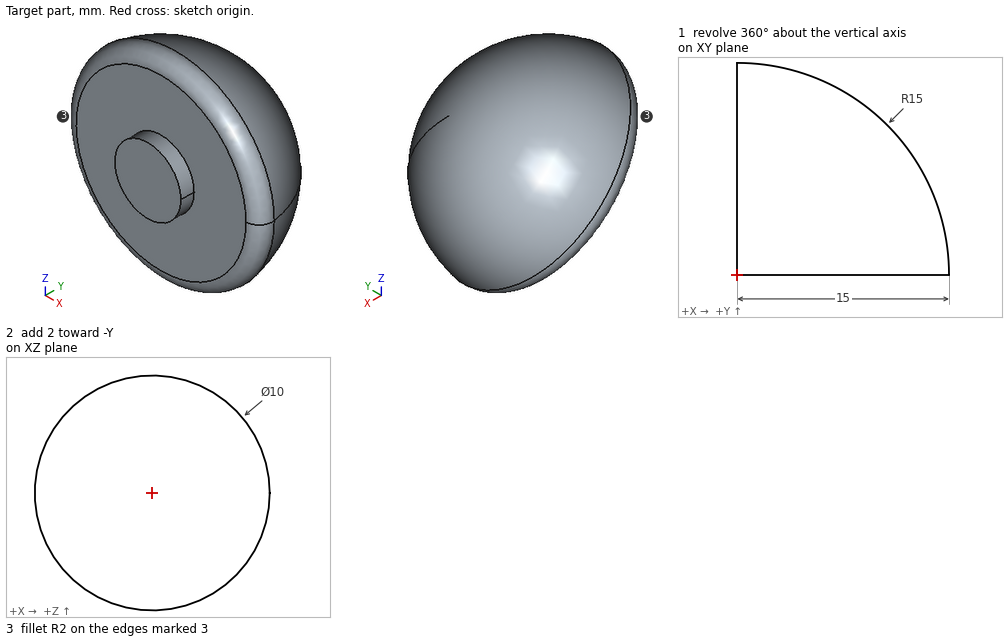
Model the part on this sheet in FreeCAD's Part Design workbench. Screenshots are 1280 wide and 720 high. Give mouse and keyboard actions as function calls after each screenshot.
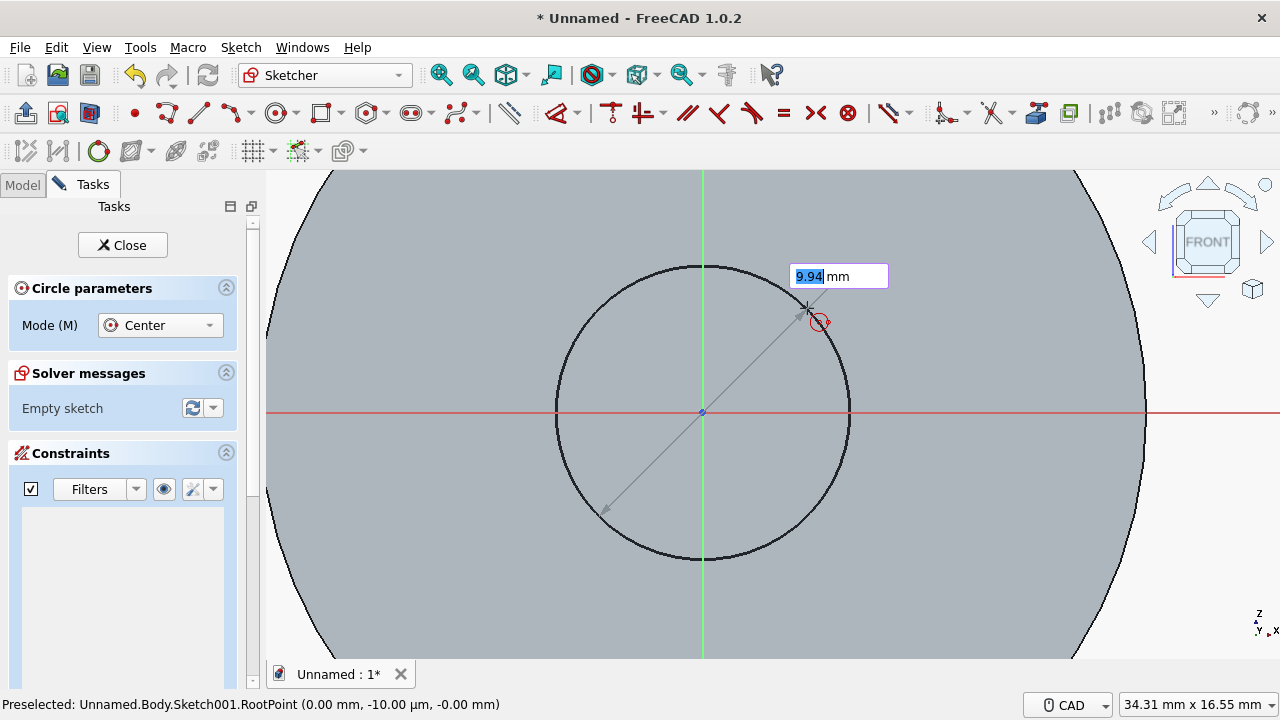
text(10)
key(Return)
key(Escape)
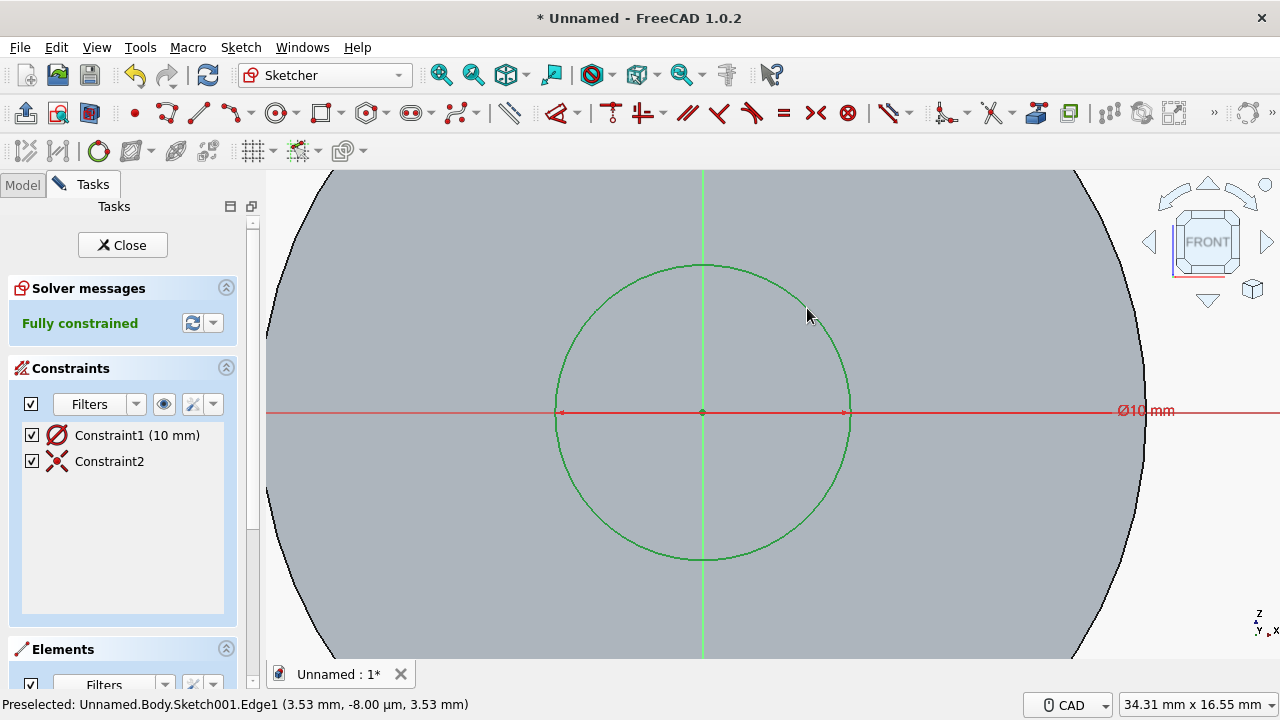
click(123, 245)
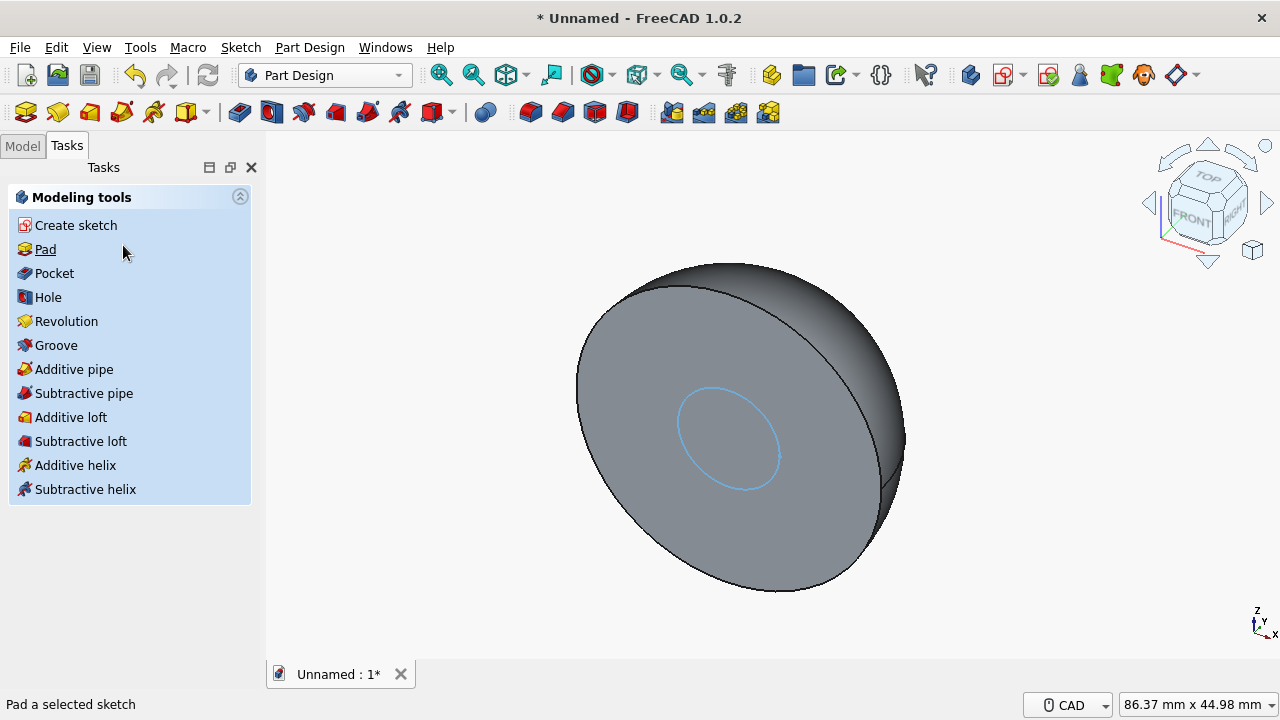
click(26, 112)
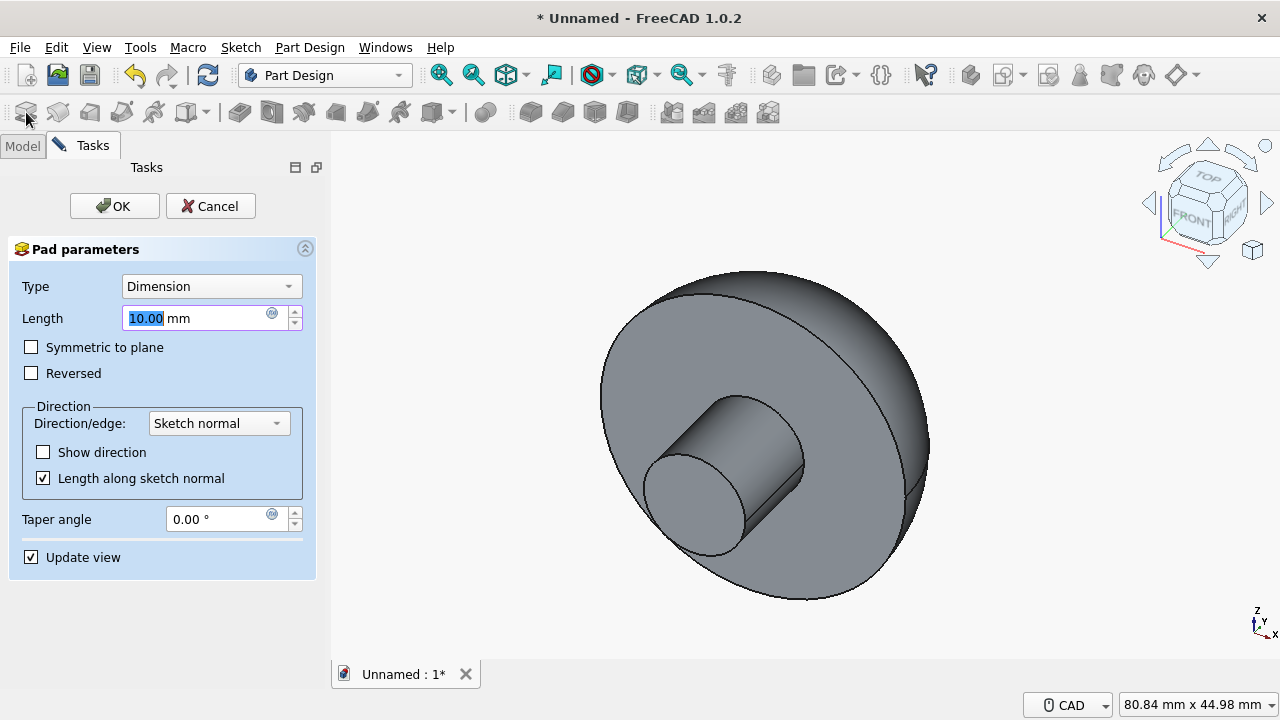
text(2)
key(Tab)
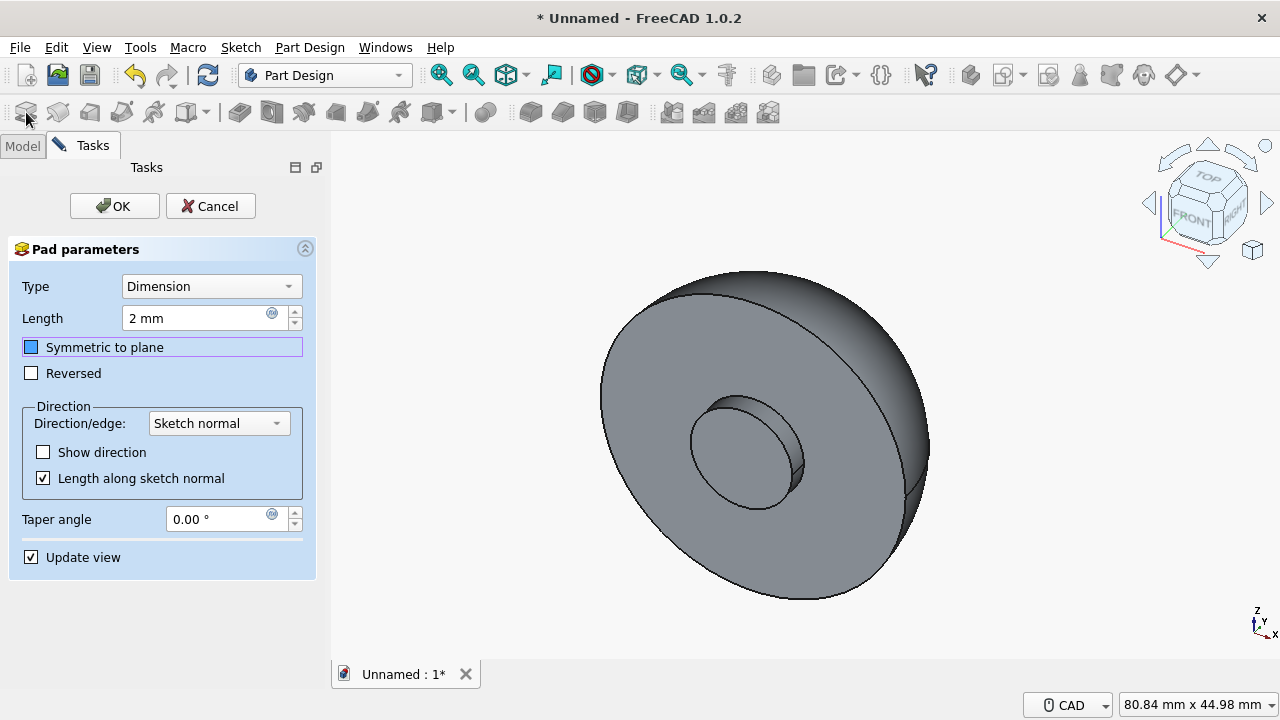
click(115, 206)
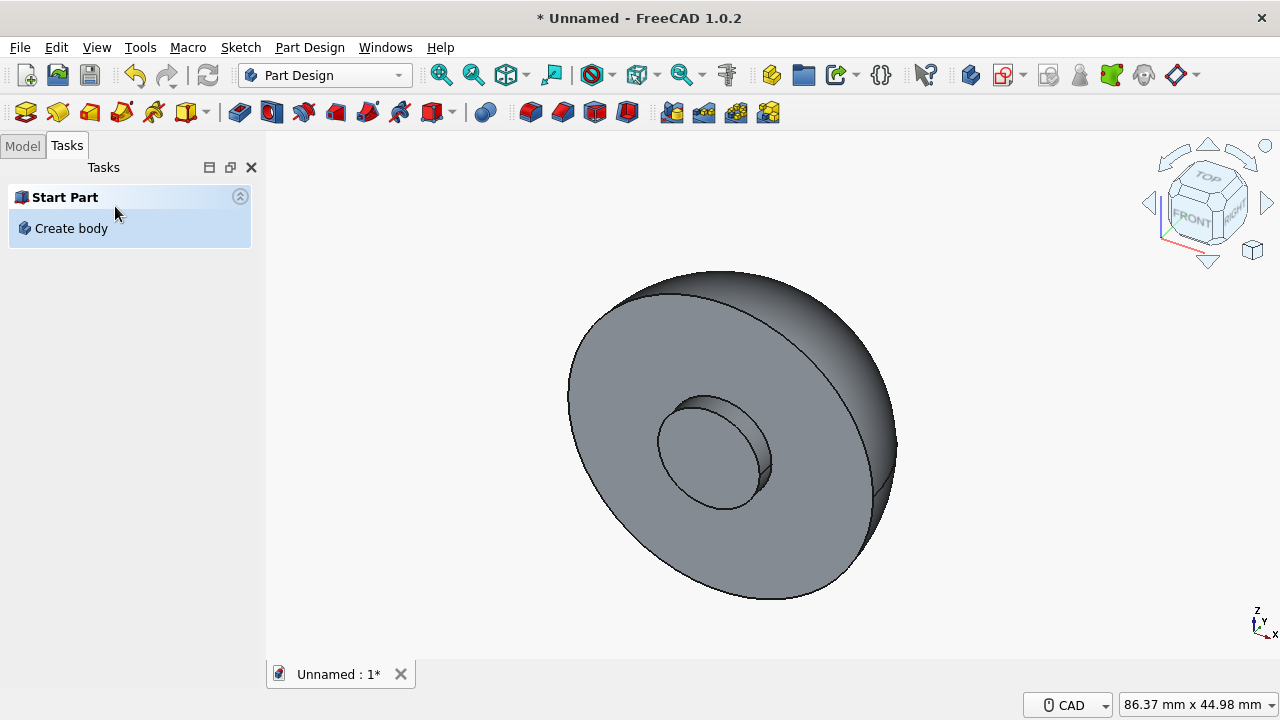
click(597, 320)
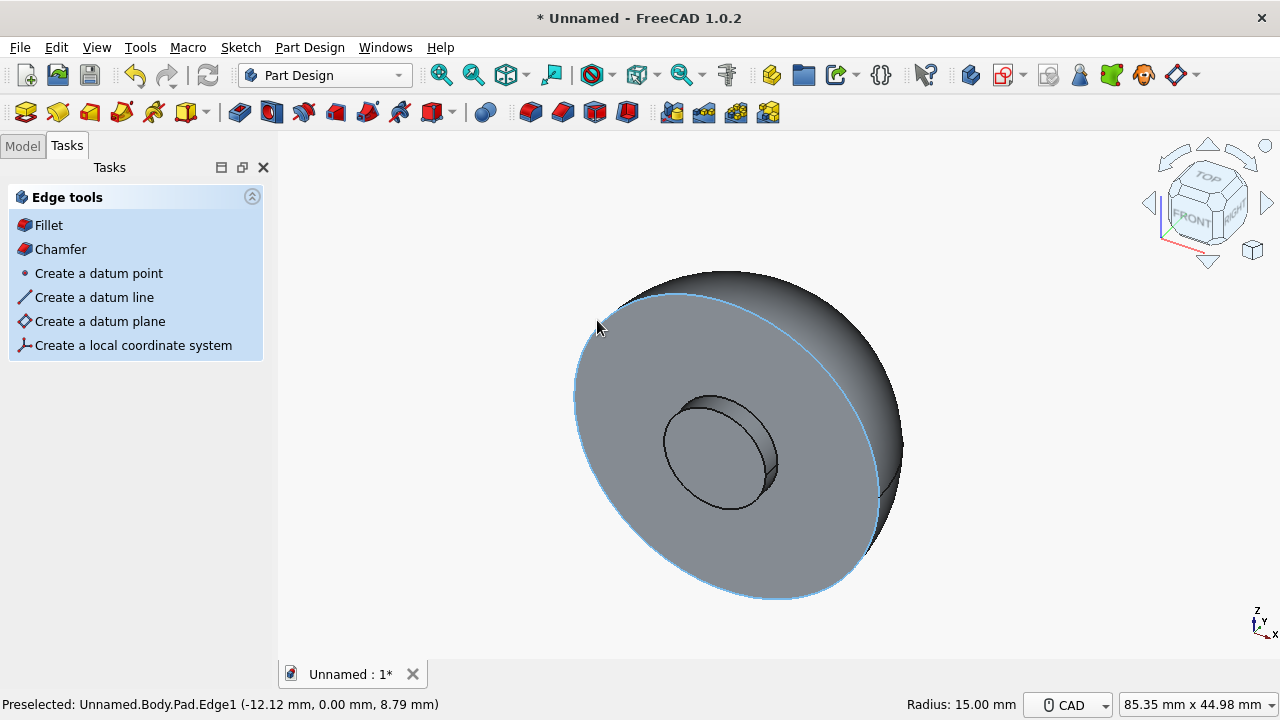
click(532, 112)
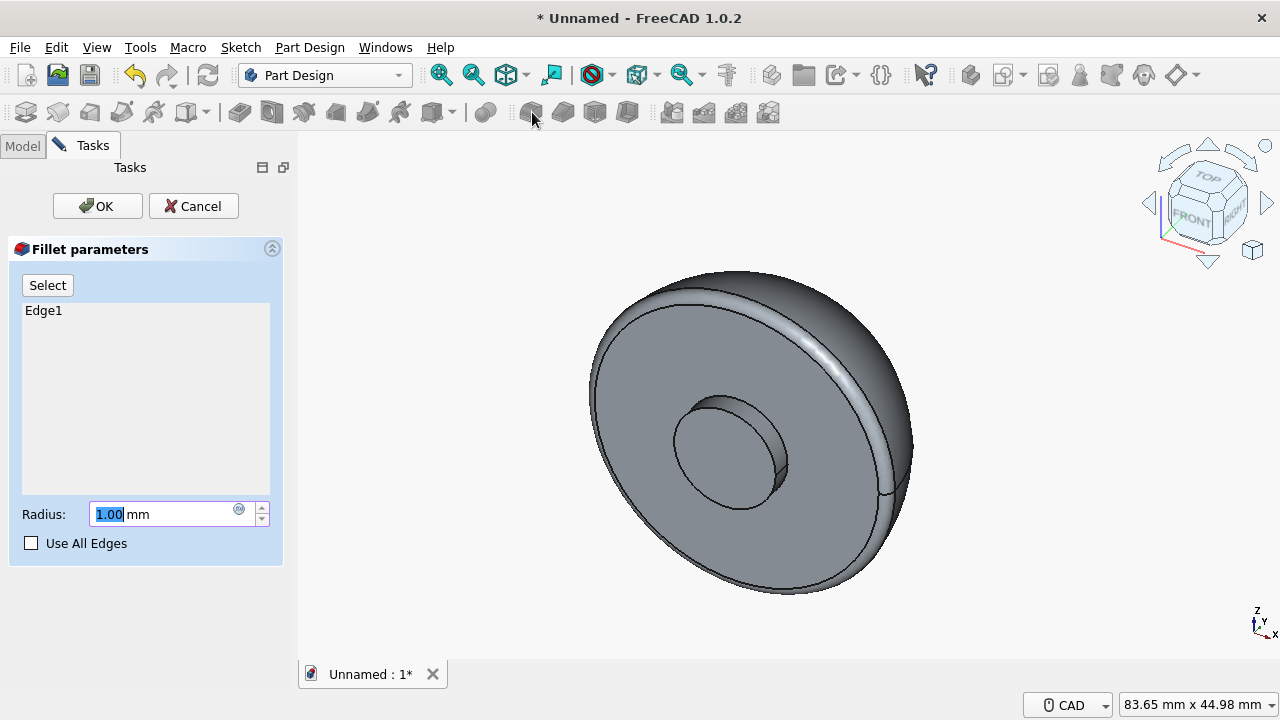
text(2)
key(Tab)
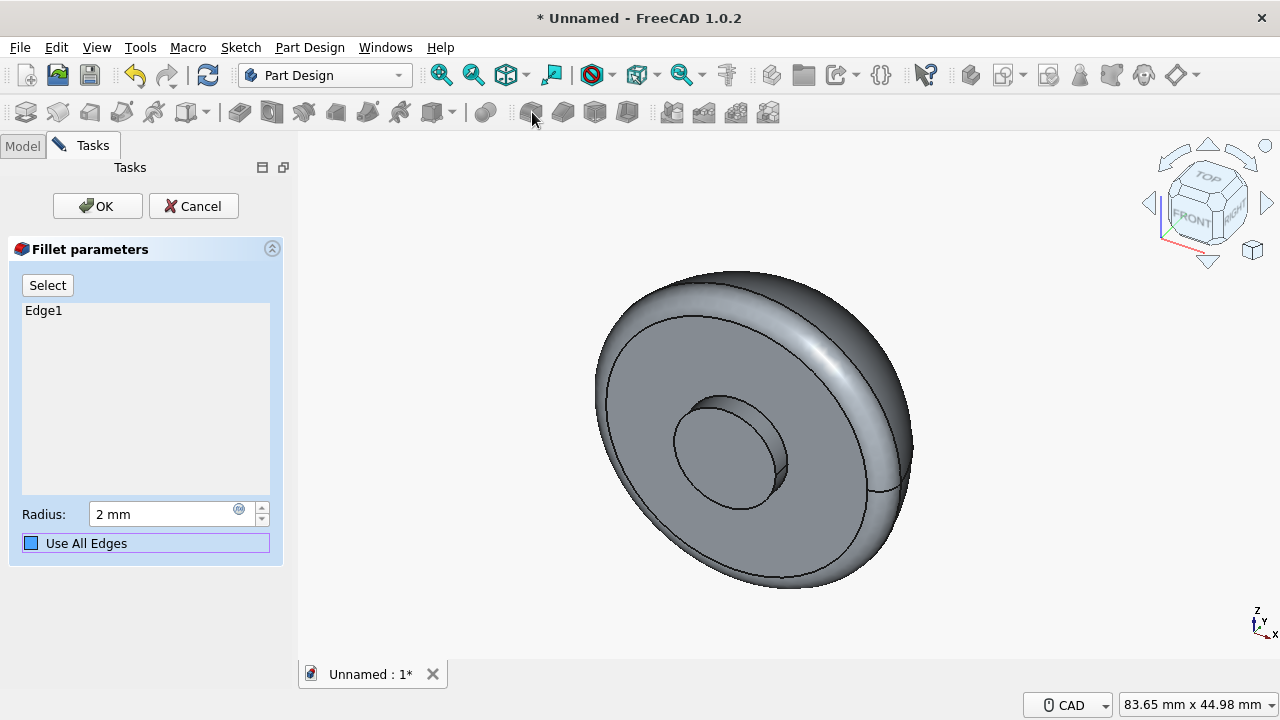
click(98, 206)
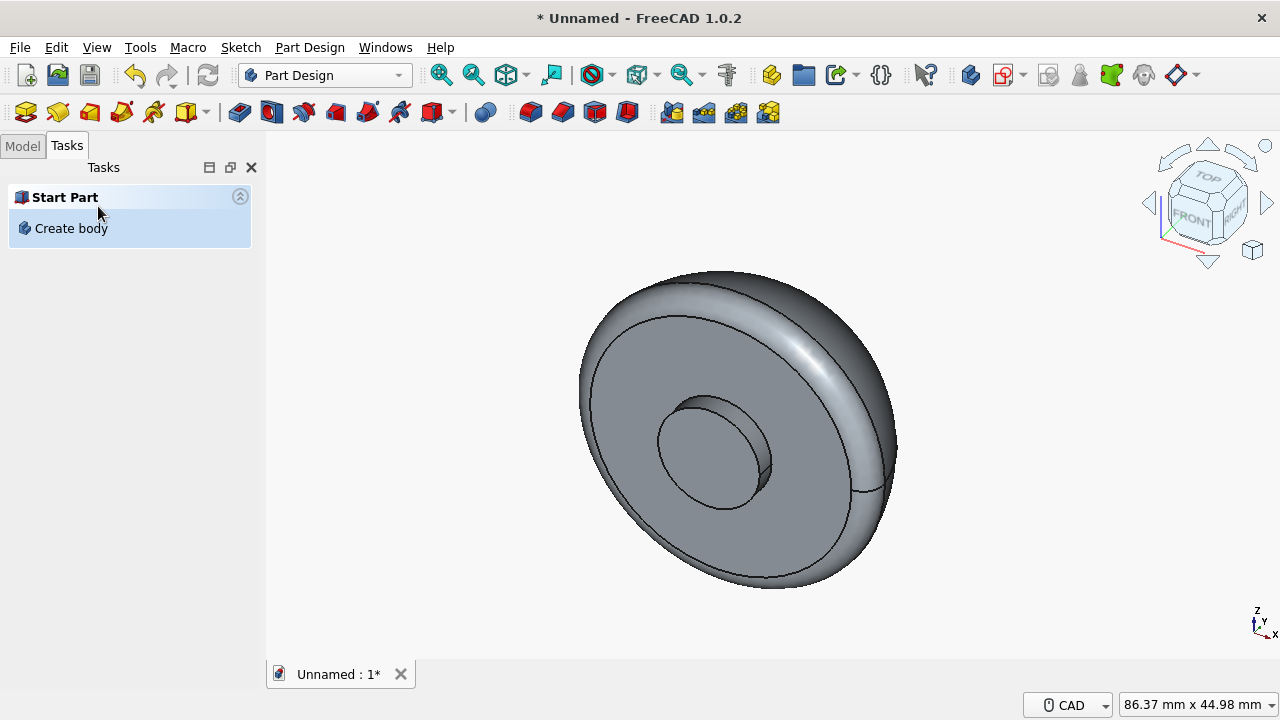
key(0)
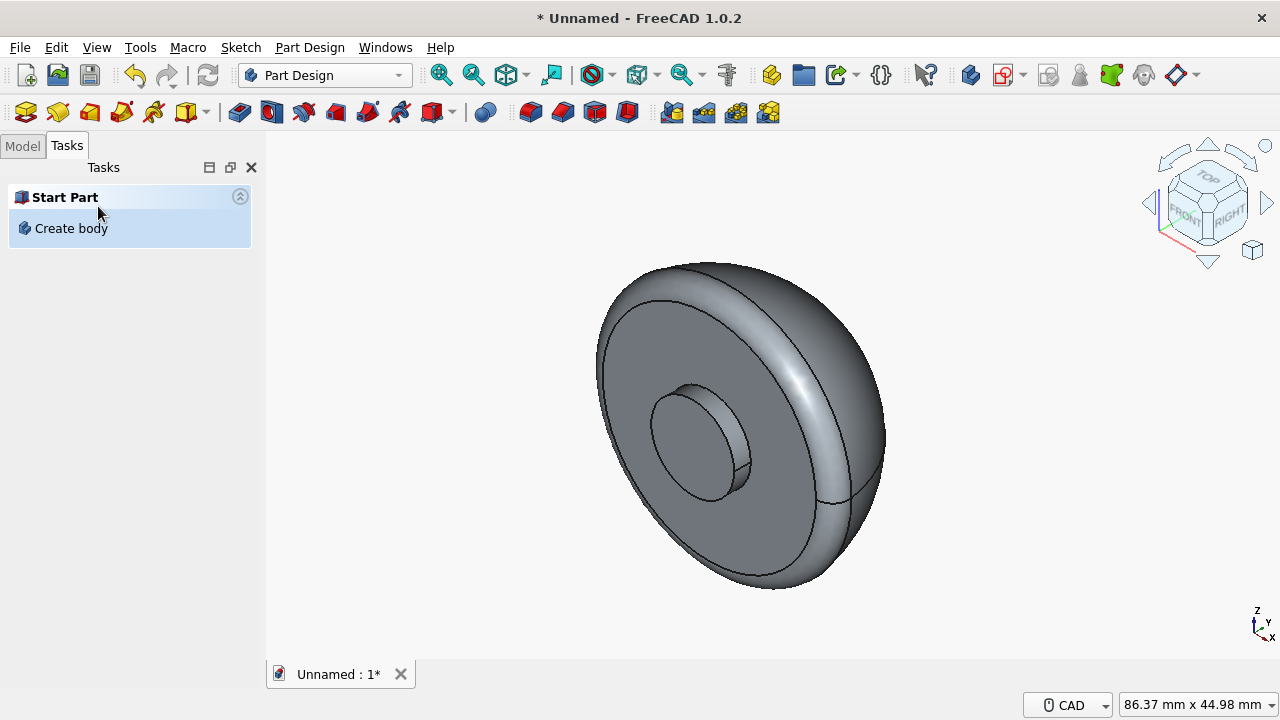
click(442, 76)